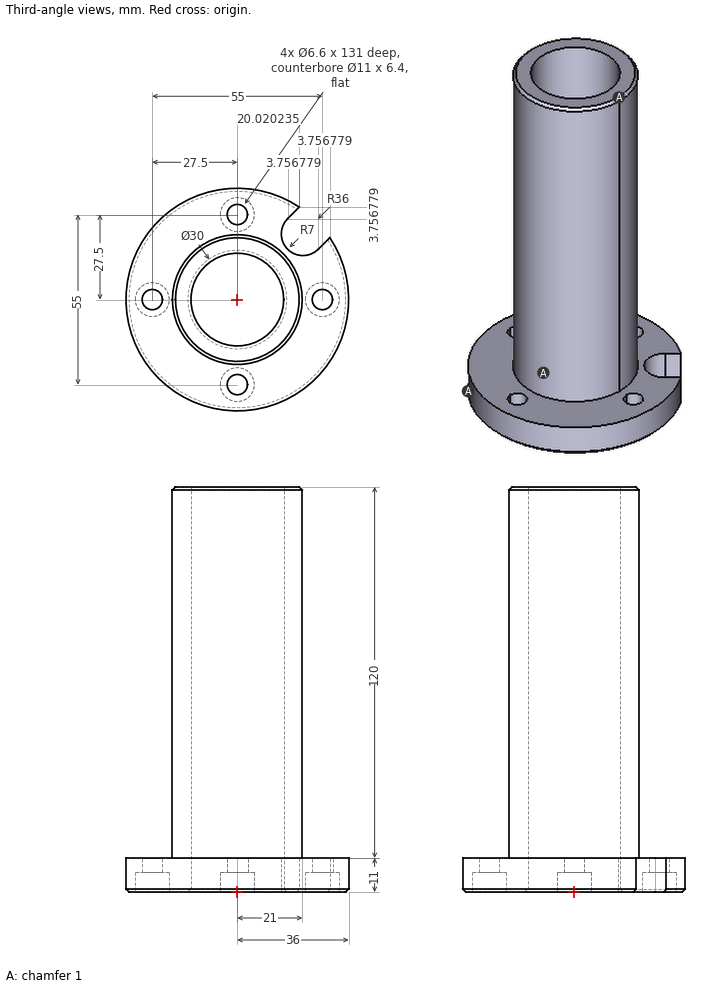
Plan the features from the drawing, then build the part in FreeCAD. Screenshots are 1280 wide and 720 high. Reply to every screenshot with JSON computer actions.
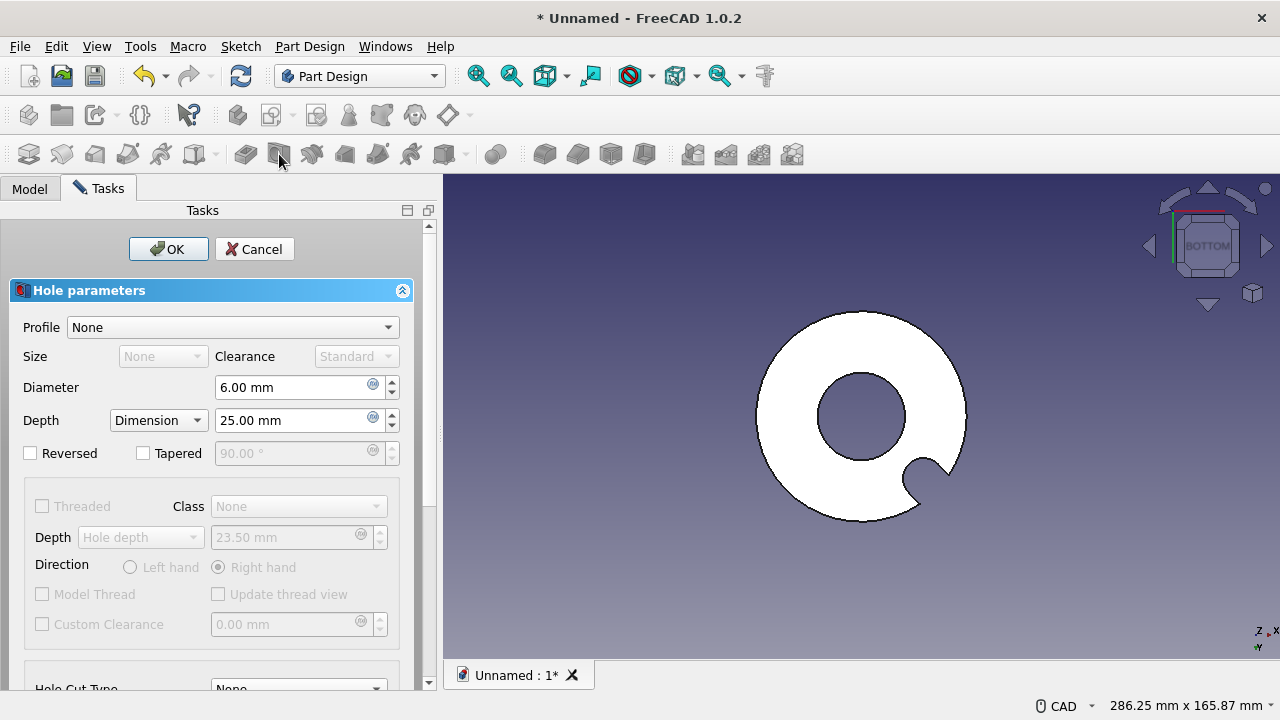
{"action": "triple_click", "coordinate": [300, 388]}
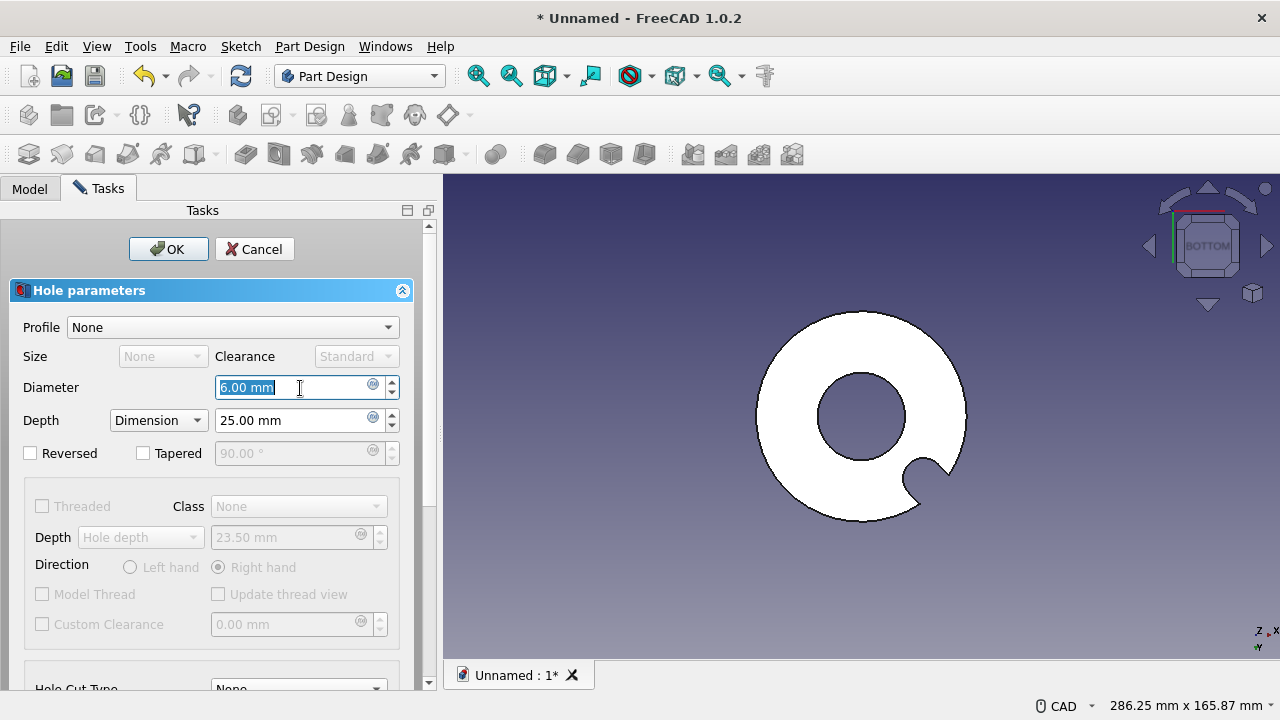
{"action": "type", "text": "6.6"}
{"action": "key", "text": "Tab"}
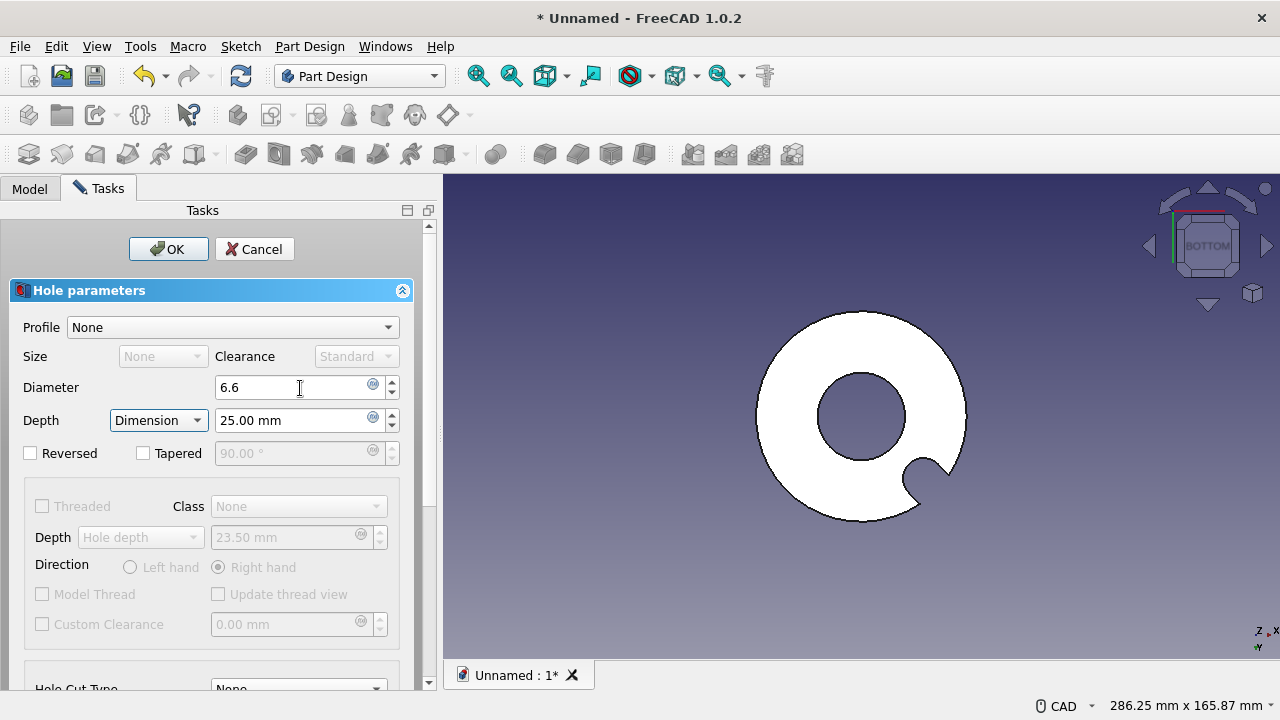
{"action": "triple_click", "coordinate": [300, 420]}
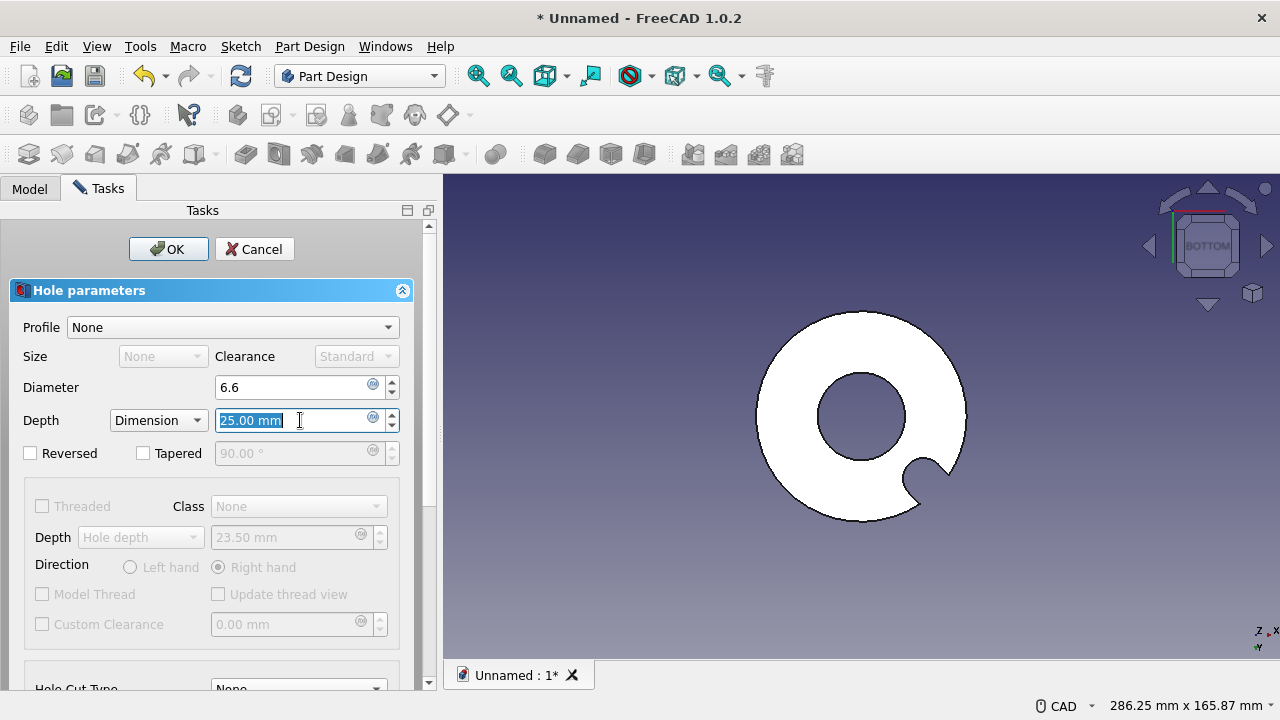
{"action": "type", "text": "131"}
{"action": "key", "text": "Tab"}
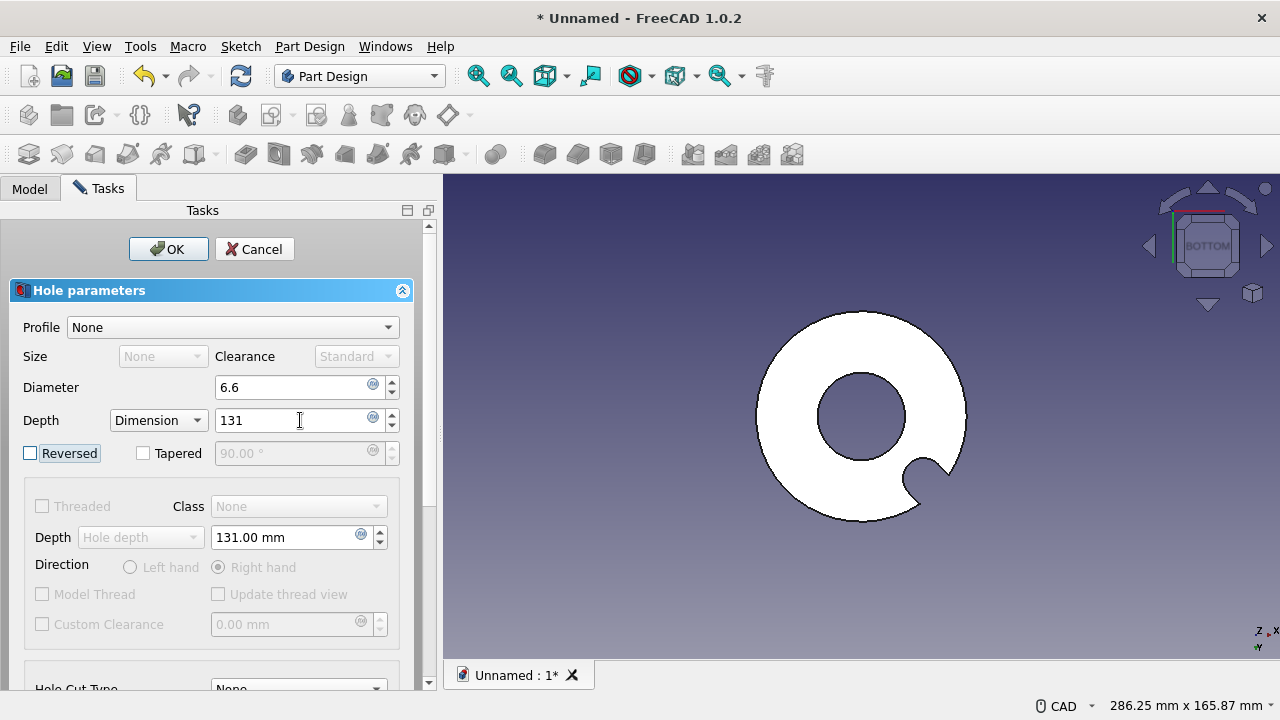
{"action": "left_click", "coordinate": [31, 453]}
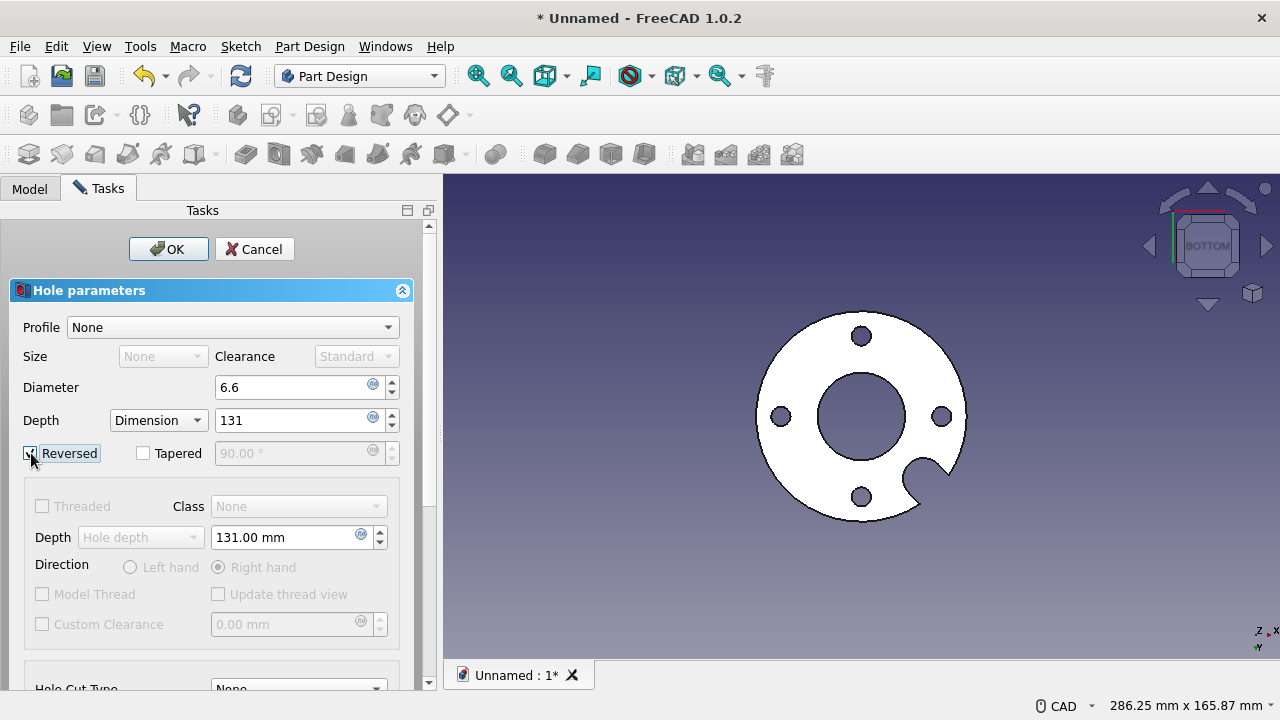
{"action": "scroll", "coordinate": [429, 455], "scroll_direction": "down", "scroll_amount": 2}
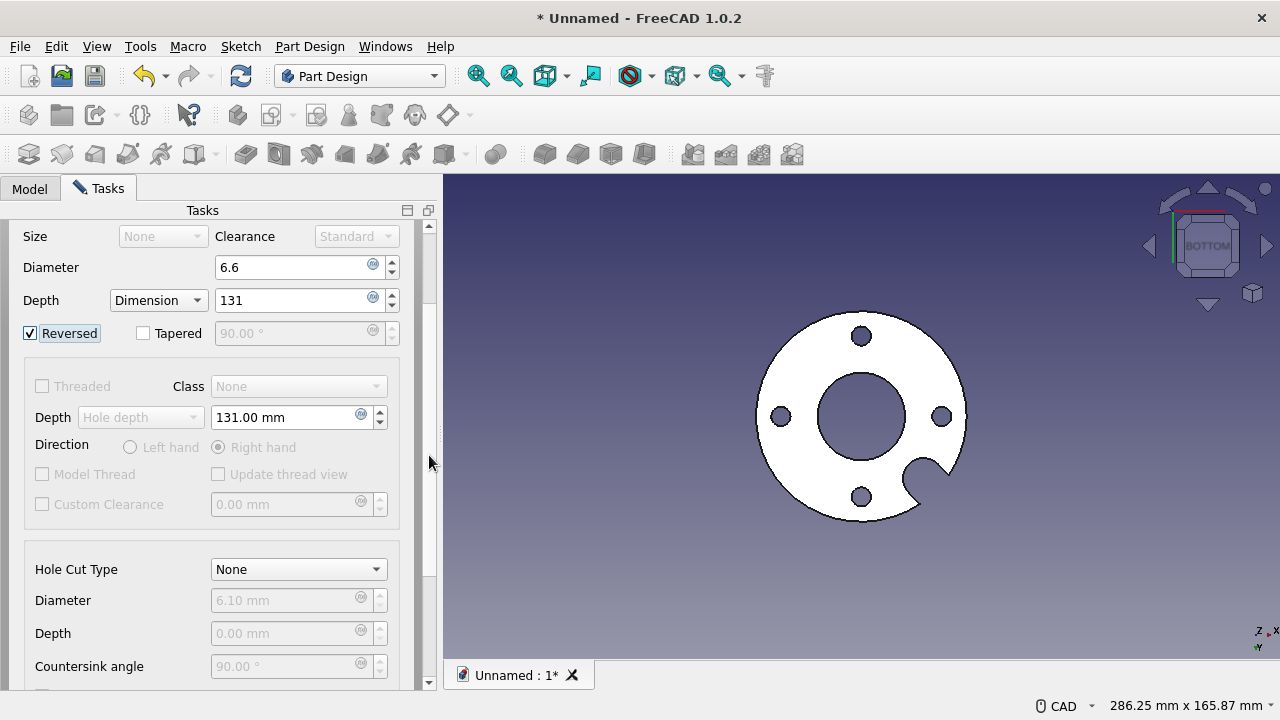
{"action": "left_click", "coordinate": [300, 570]}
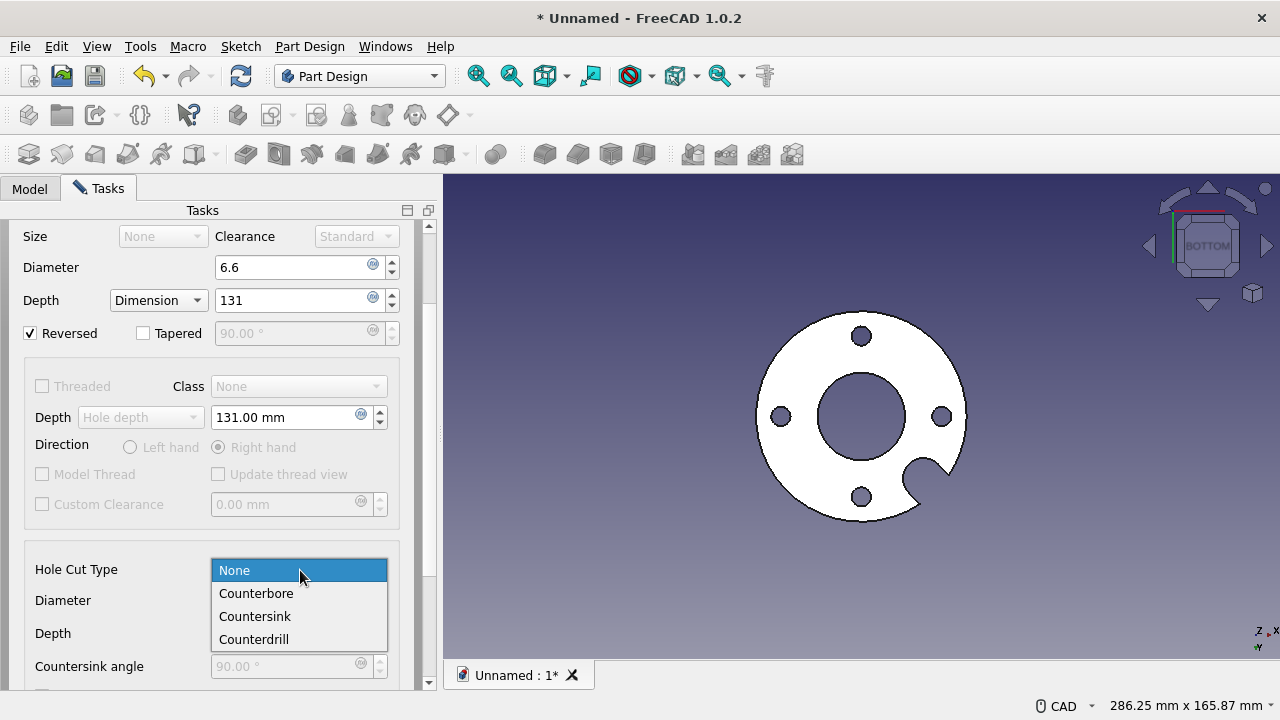
{"action": "left_click", "coordinate": [298, 594]}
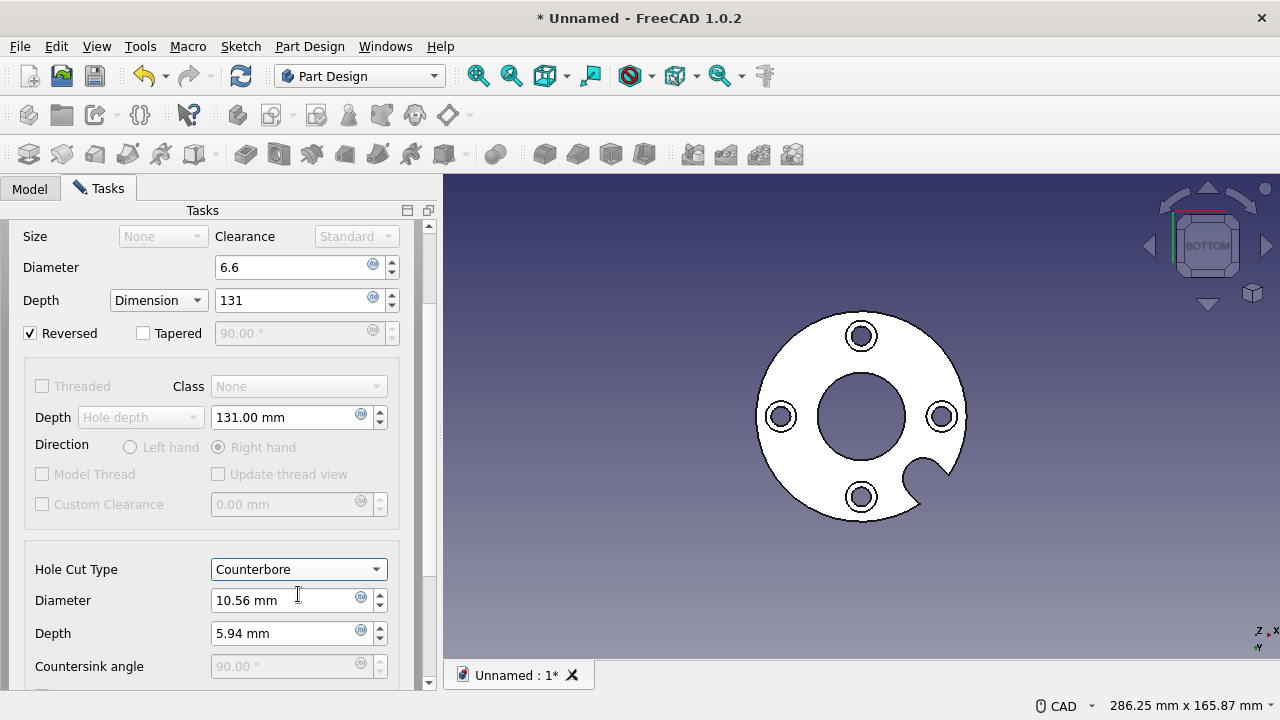
{"action": "triple_click", "coordinate": [292, 600]}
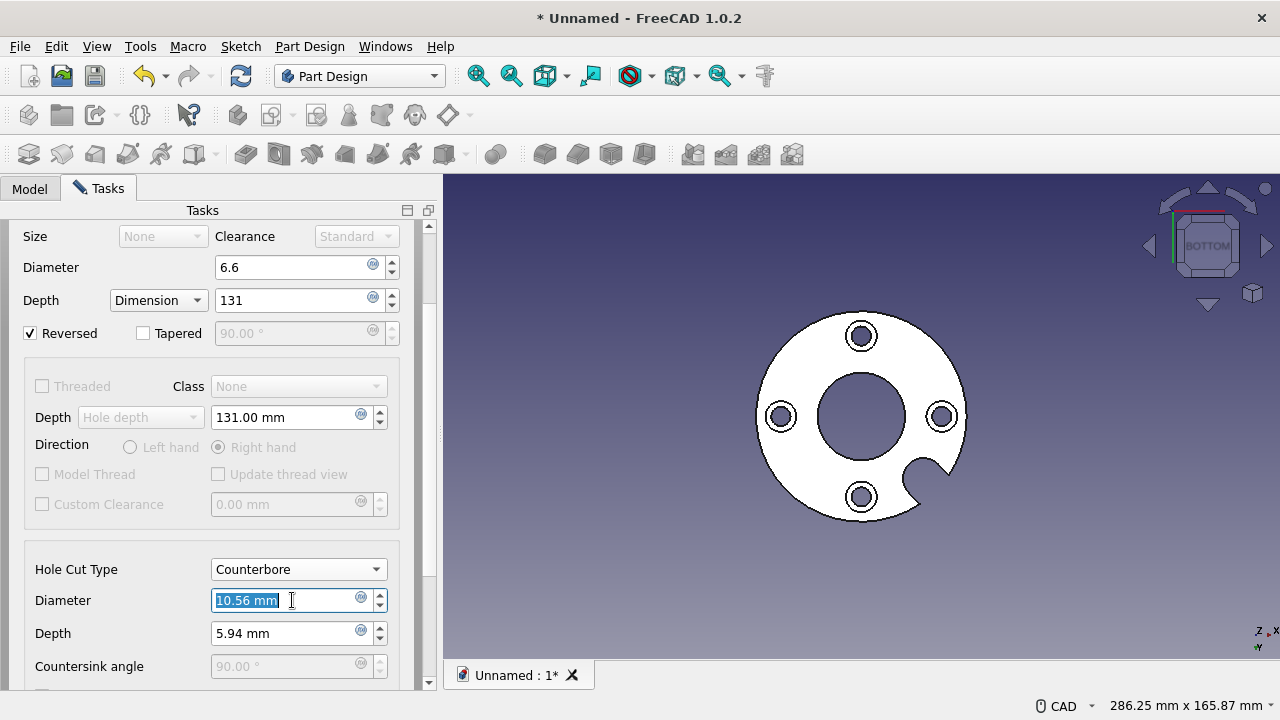
{"action": "type", "text": "11"}
{"action": "key", "text": "Tab"}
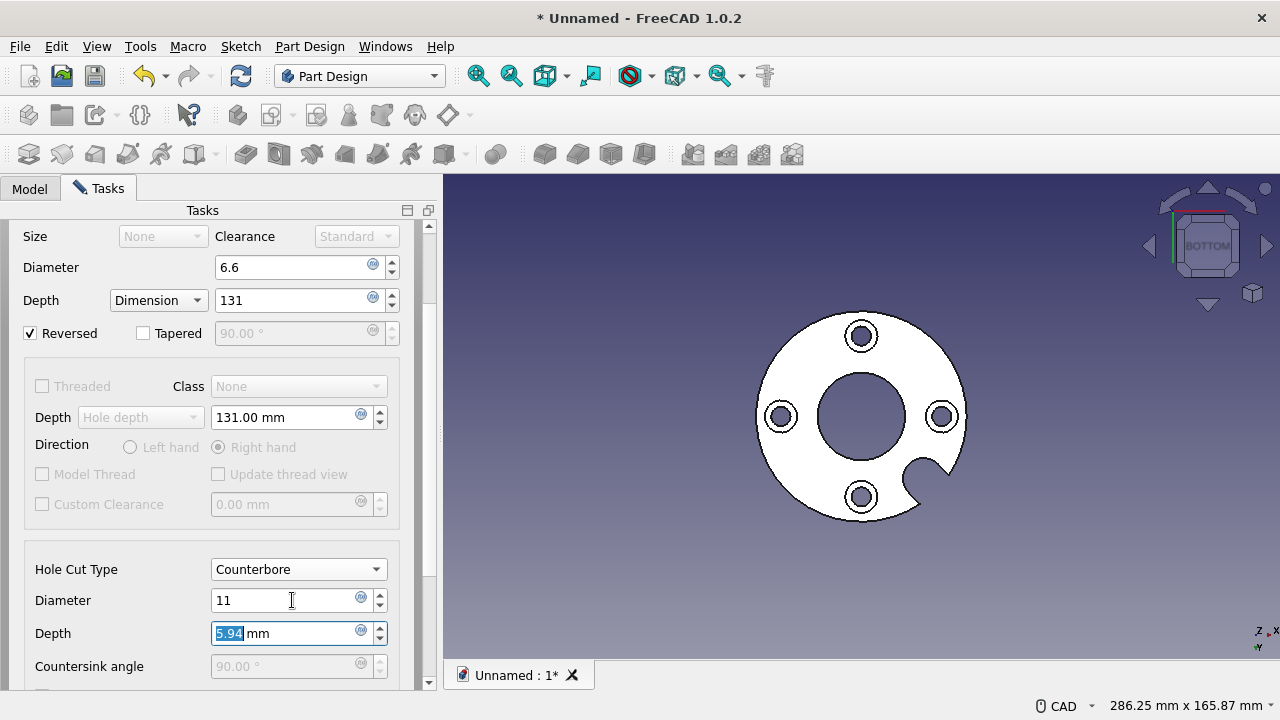
{"action": "type", "text": "6.4"}
{"action": "key", "text": "Tab"}